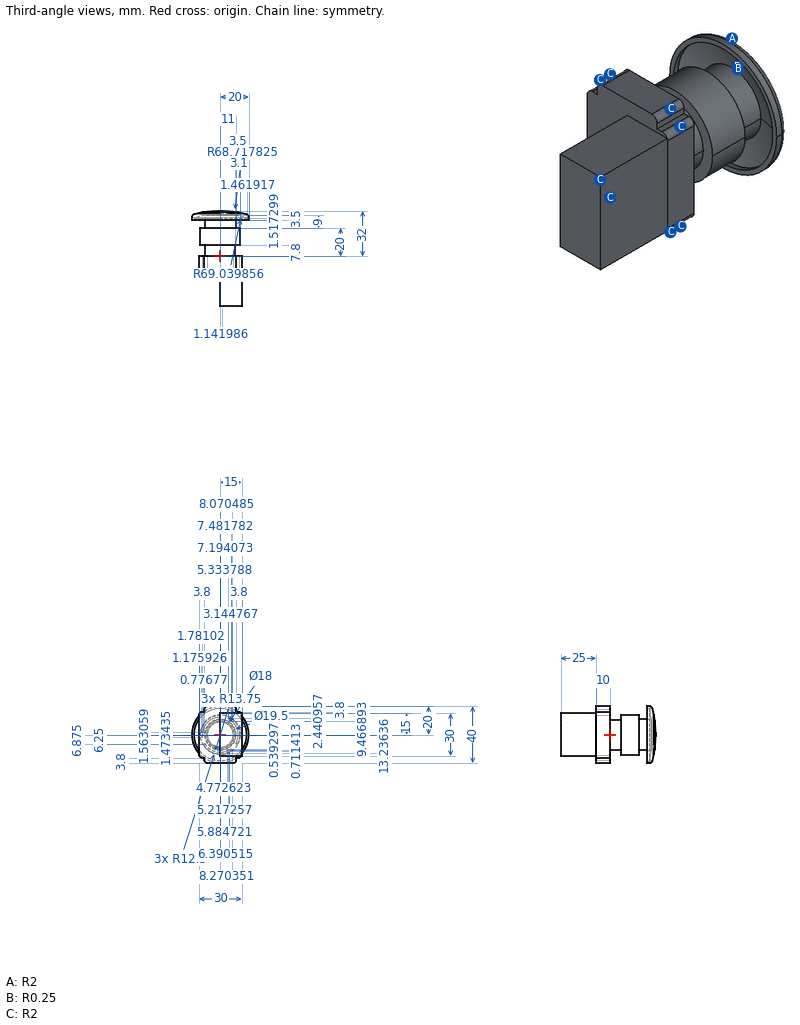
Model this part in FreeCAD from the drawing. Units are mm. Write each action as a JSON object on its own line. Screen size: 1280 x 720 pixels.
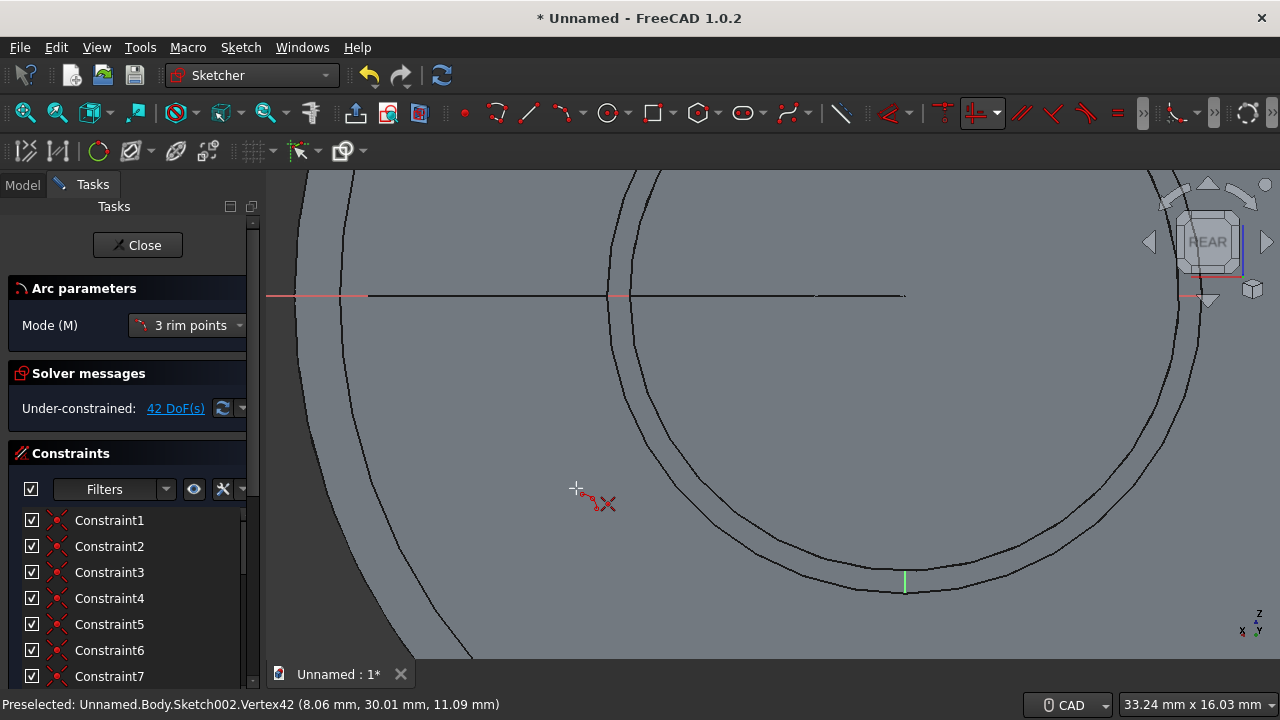
{"action": "left_click", "coordinate": [575, 489]}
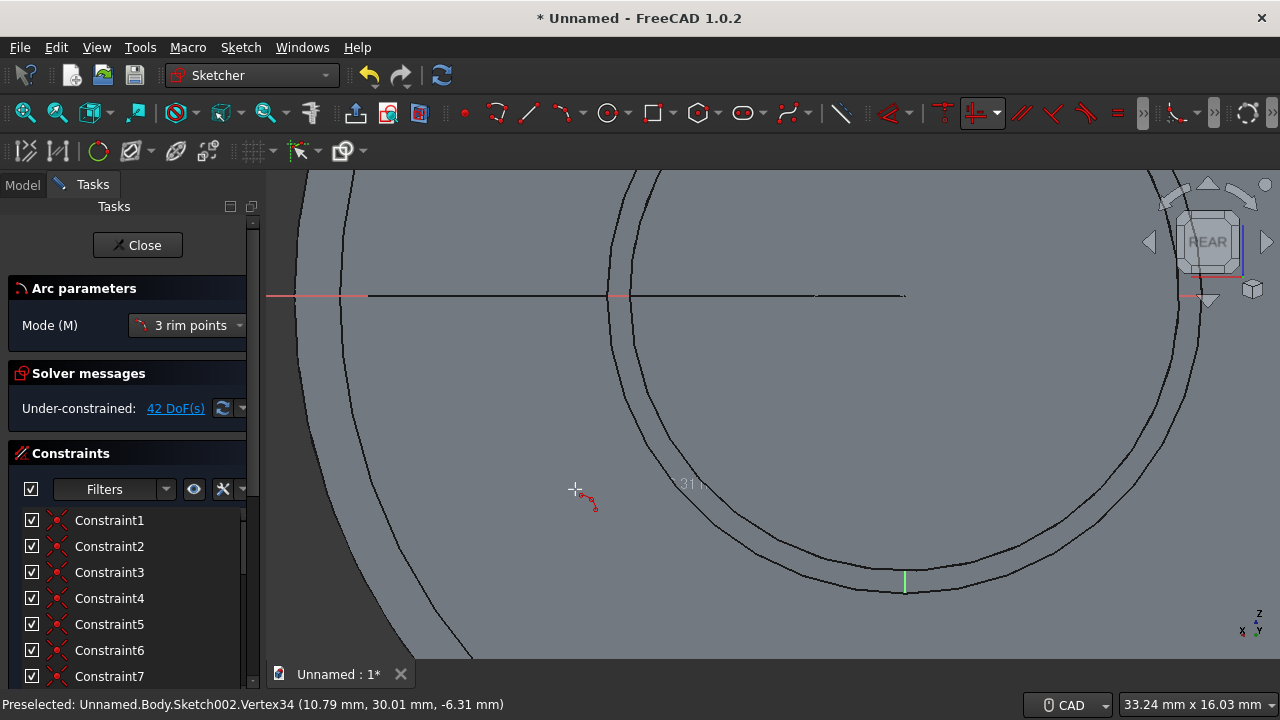
{"action": "scroll", "coordinate": [576, 488], "scroll_direction": "down", "scroll_amount": 5}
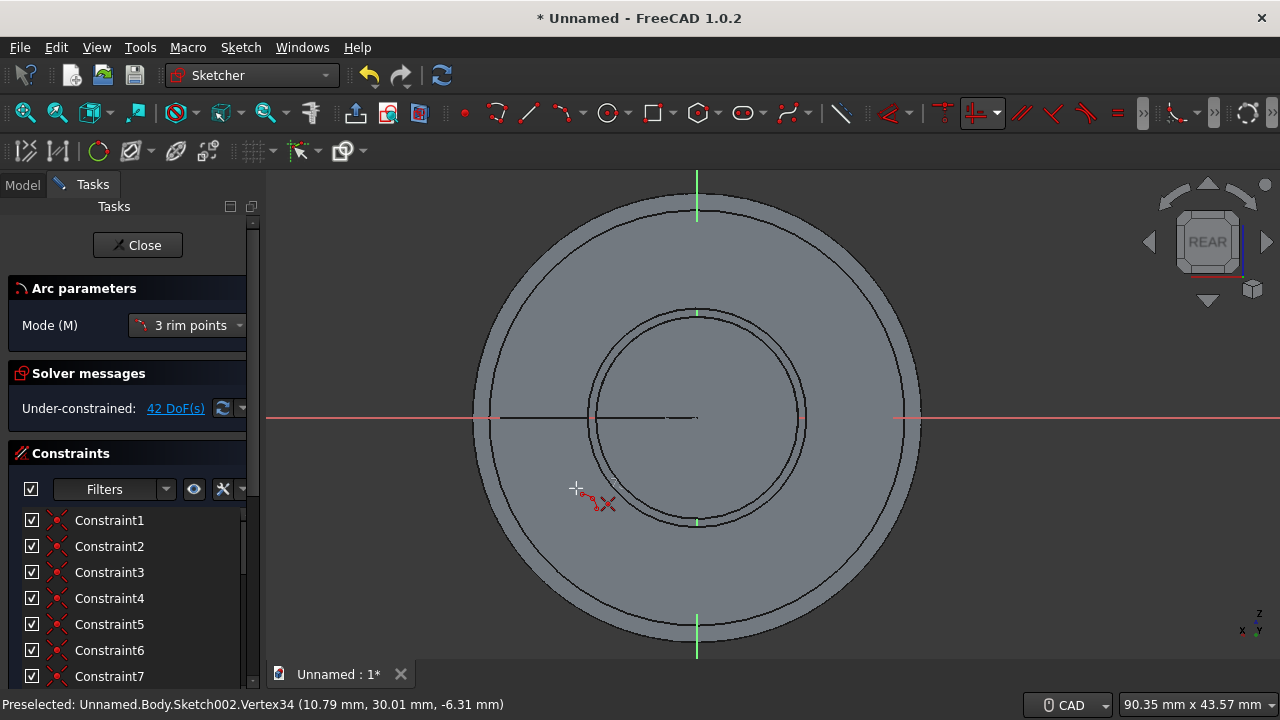
{"action": "scroll", "coordinate": [613, 305], "scroll_direction": "up", "scroll_amount": 8}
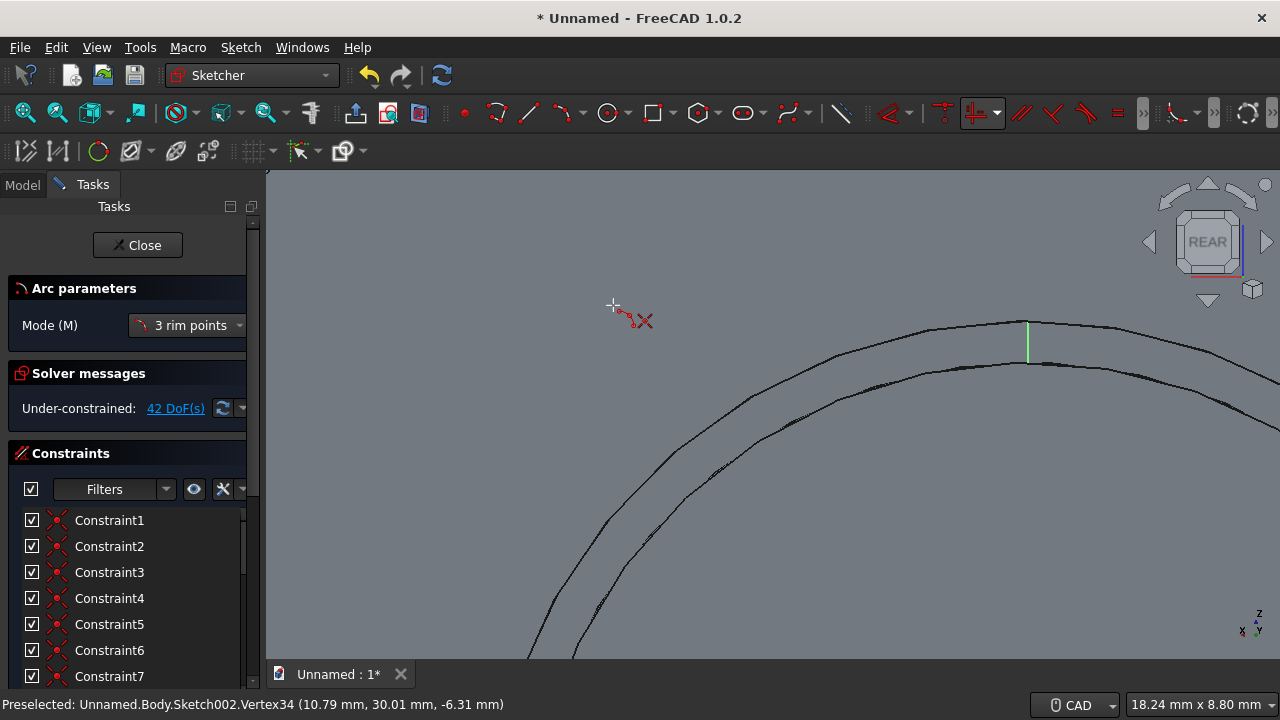
{"action": "left_click", "coordinate": [612, 312]}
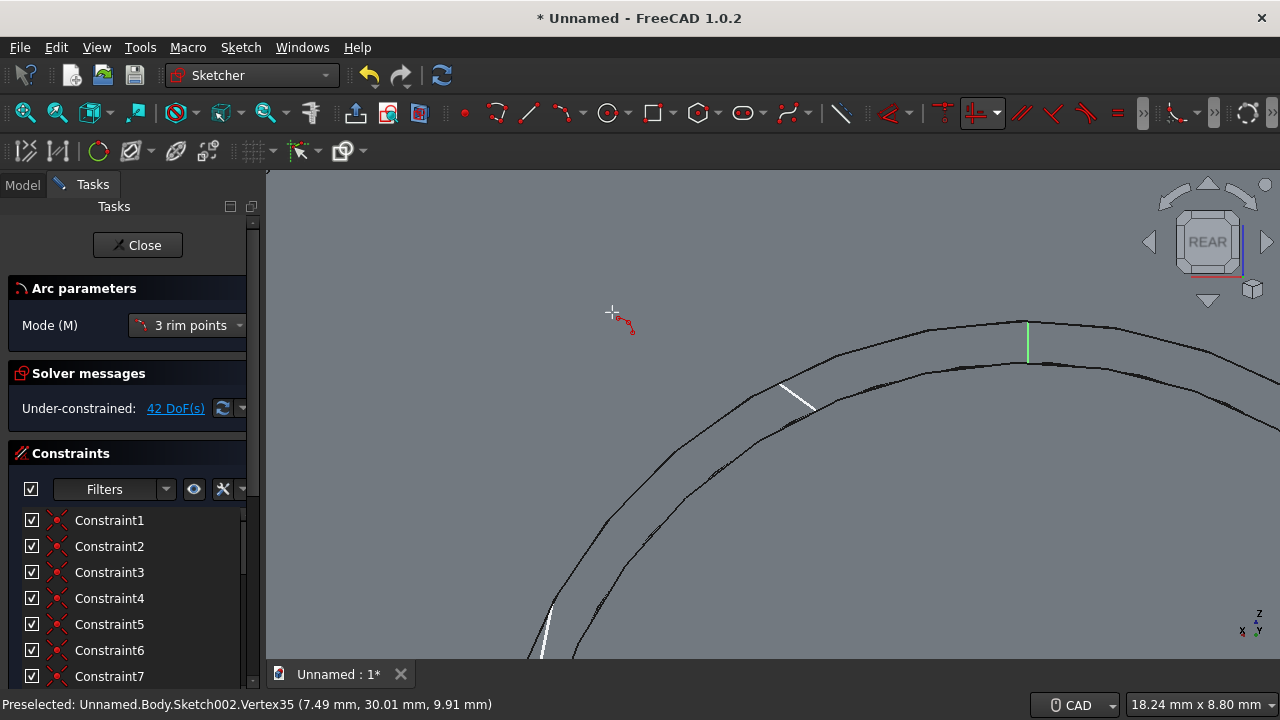
{"action": "scroll", "coordinate": [613, 305], "scroll_direction": "down", "scroll_amount": 8}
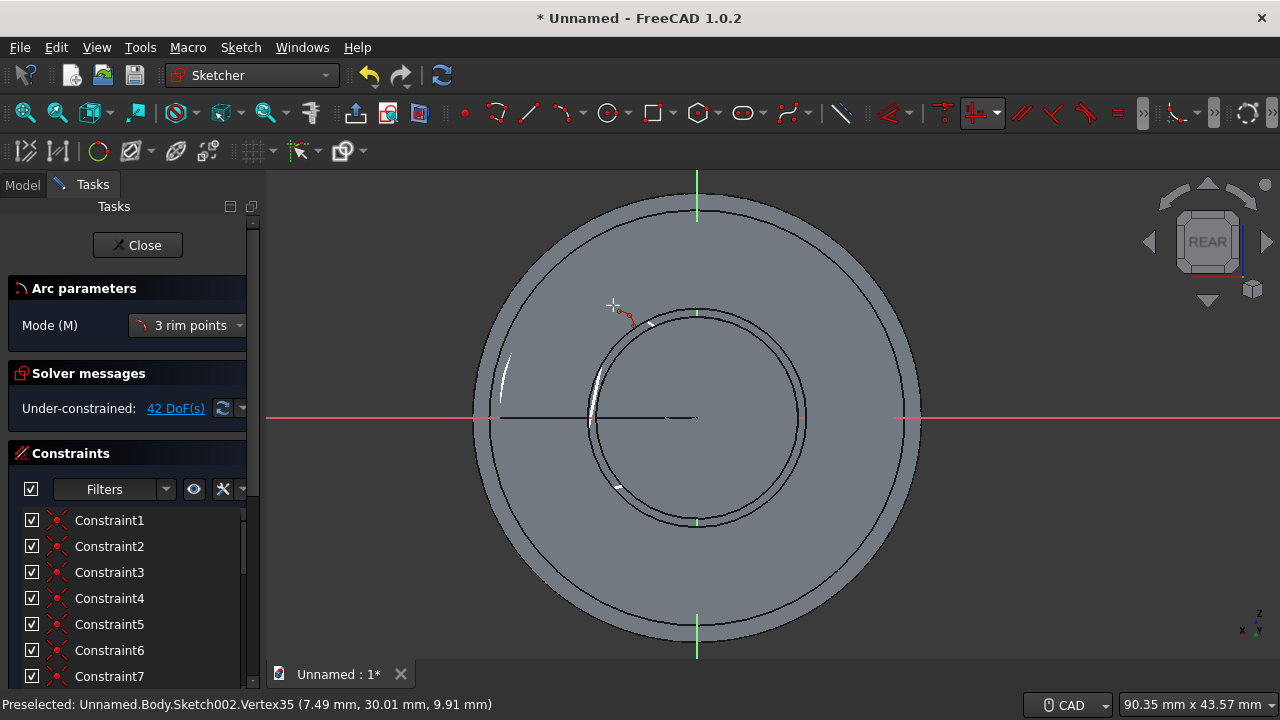
{"action": "left_click", "coordinate": [560, 390]}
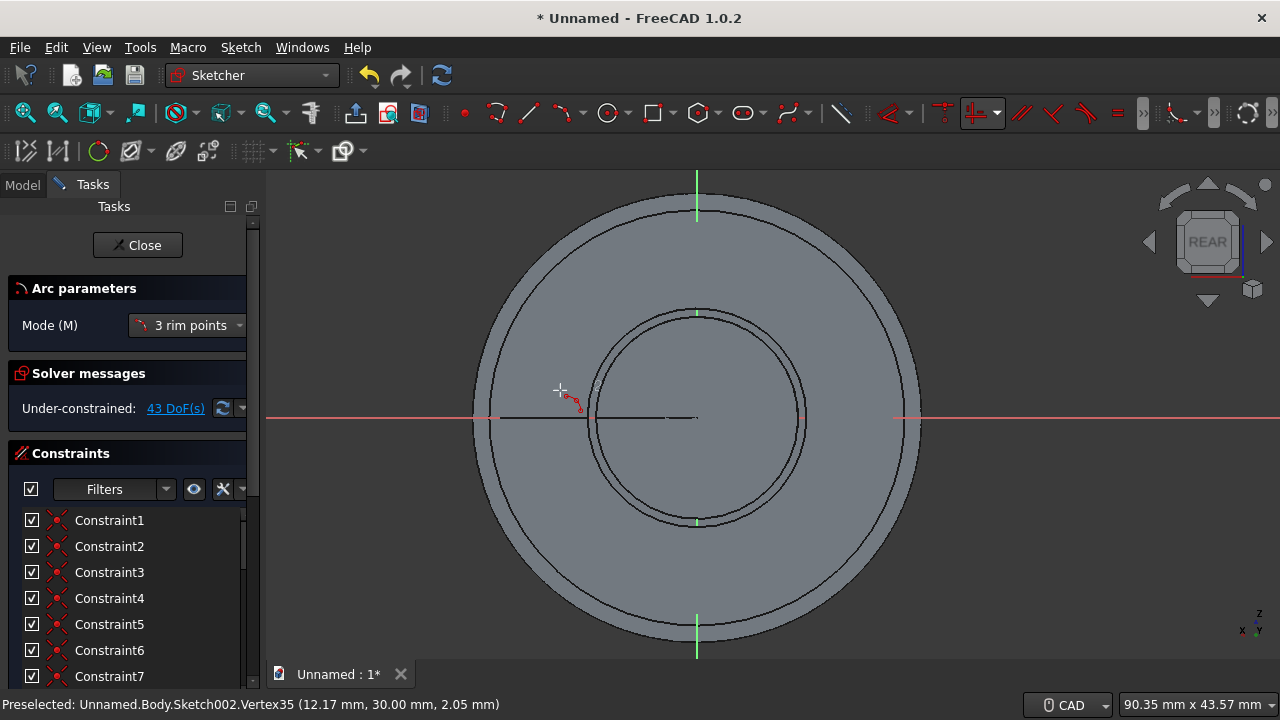
{"action": "scroll", "coordinate": [606, 293], "scroll_direction": "up", "scroll_amount": 6}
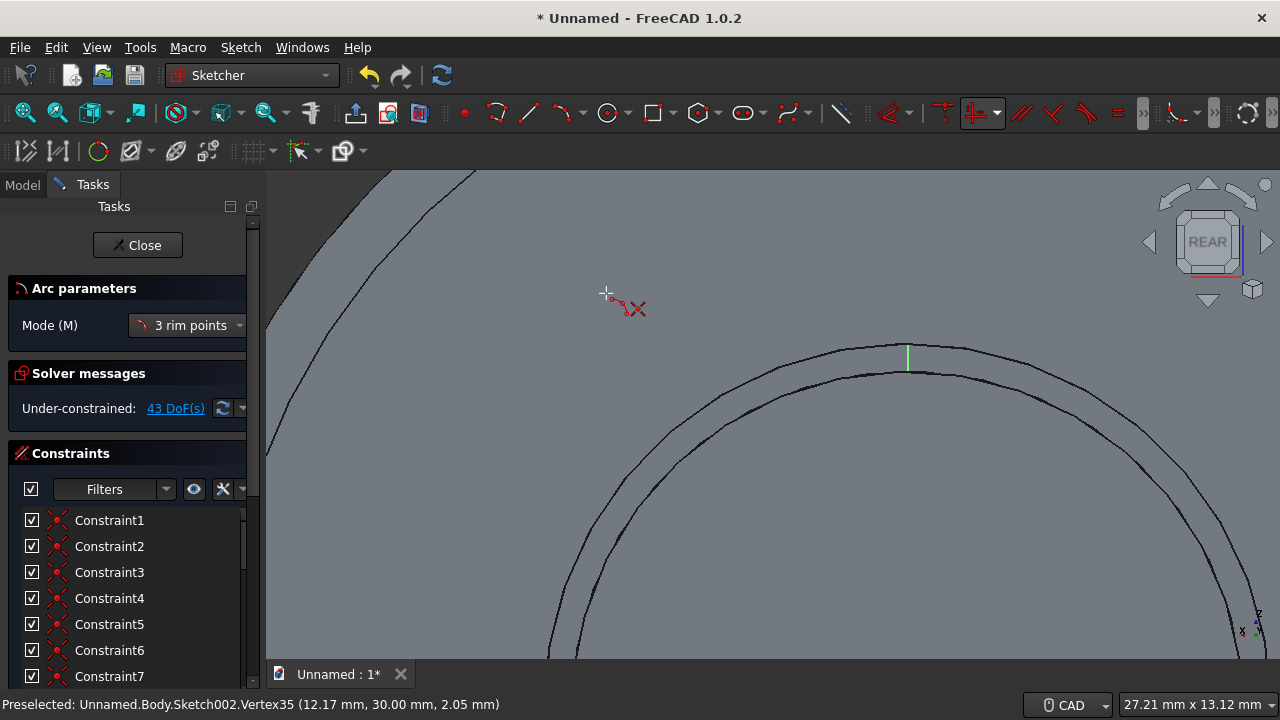
{"action": "left_click", "coordinate": [607, 294]}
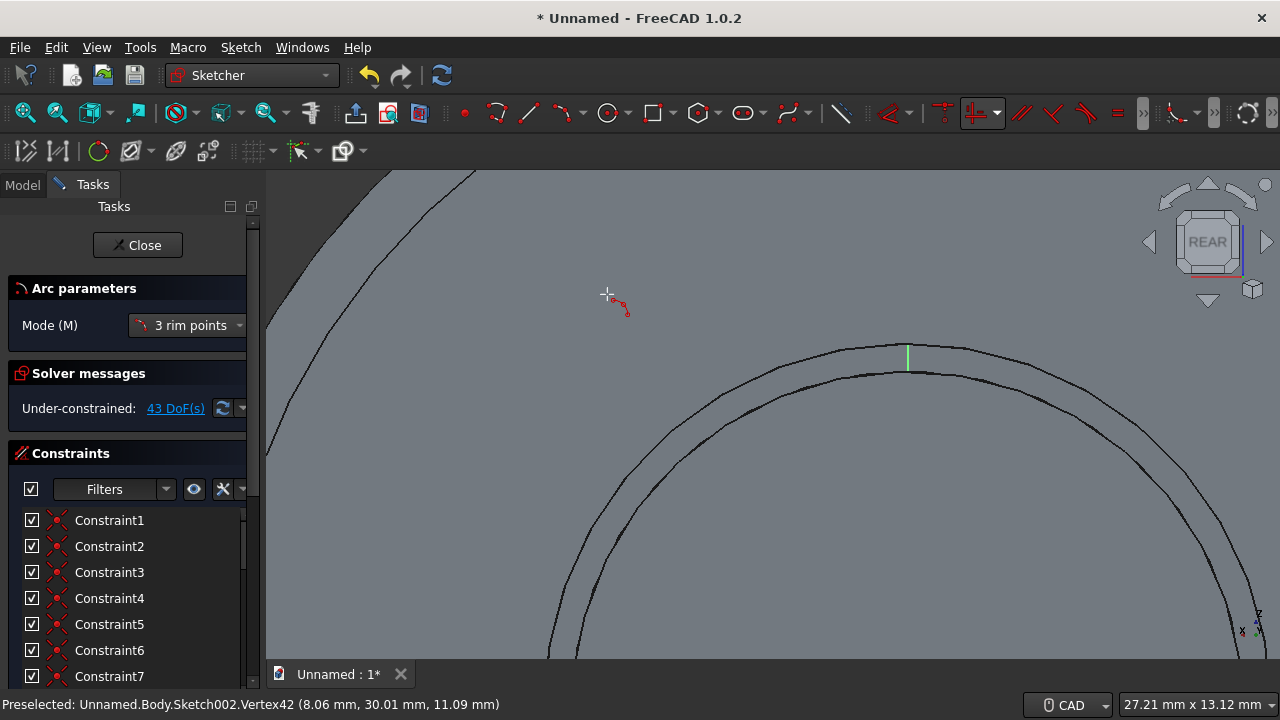
{"action": "scroll", "coordinate": [606, 293], "scroll_direction": "down", "scroll_amount": 6}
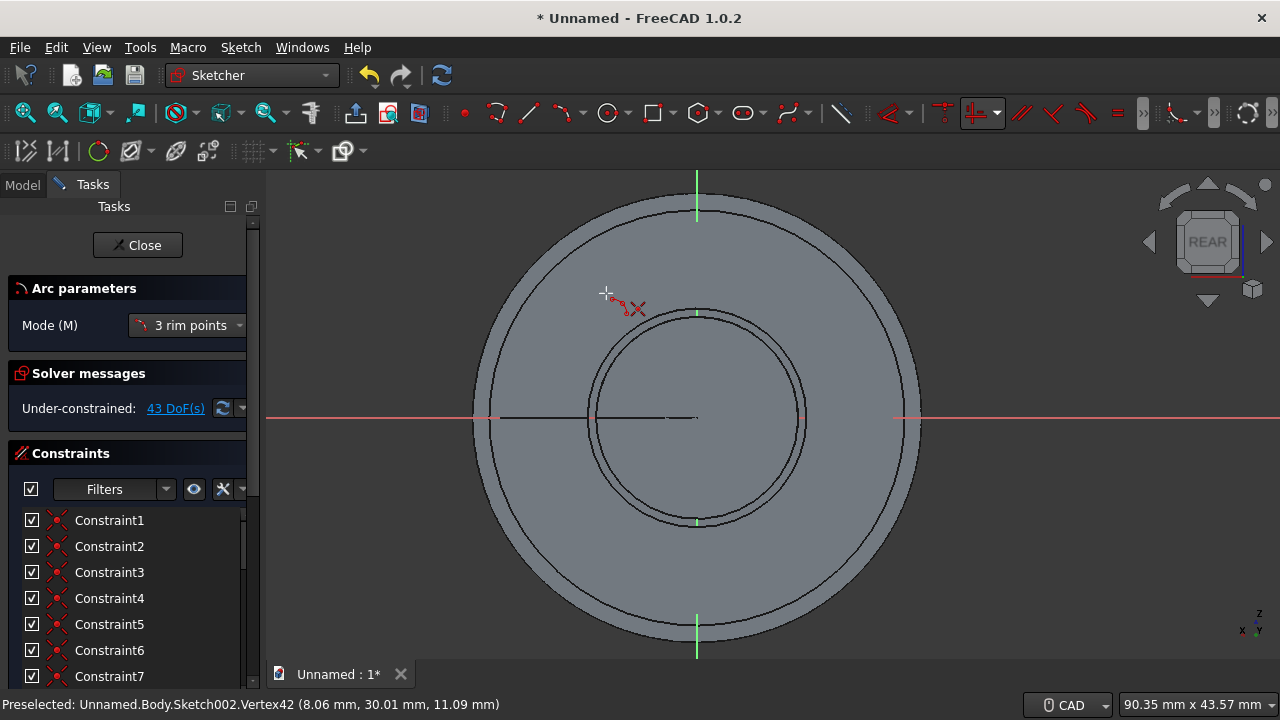
{"action": "scroll", "coordinate": [563, 495], "scroll_direction": "up", "scroll_amount": 5}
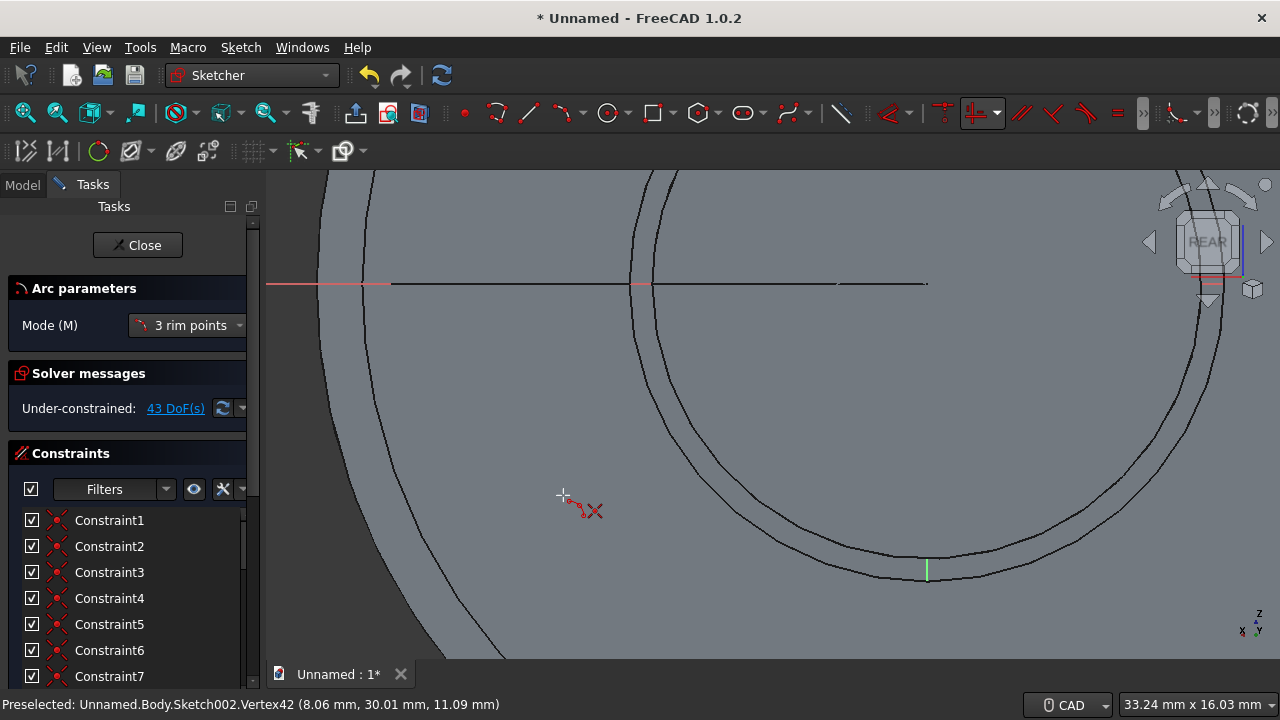
{"action": "left_click", "coordinate": [562, 496]}